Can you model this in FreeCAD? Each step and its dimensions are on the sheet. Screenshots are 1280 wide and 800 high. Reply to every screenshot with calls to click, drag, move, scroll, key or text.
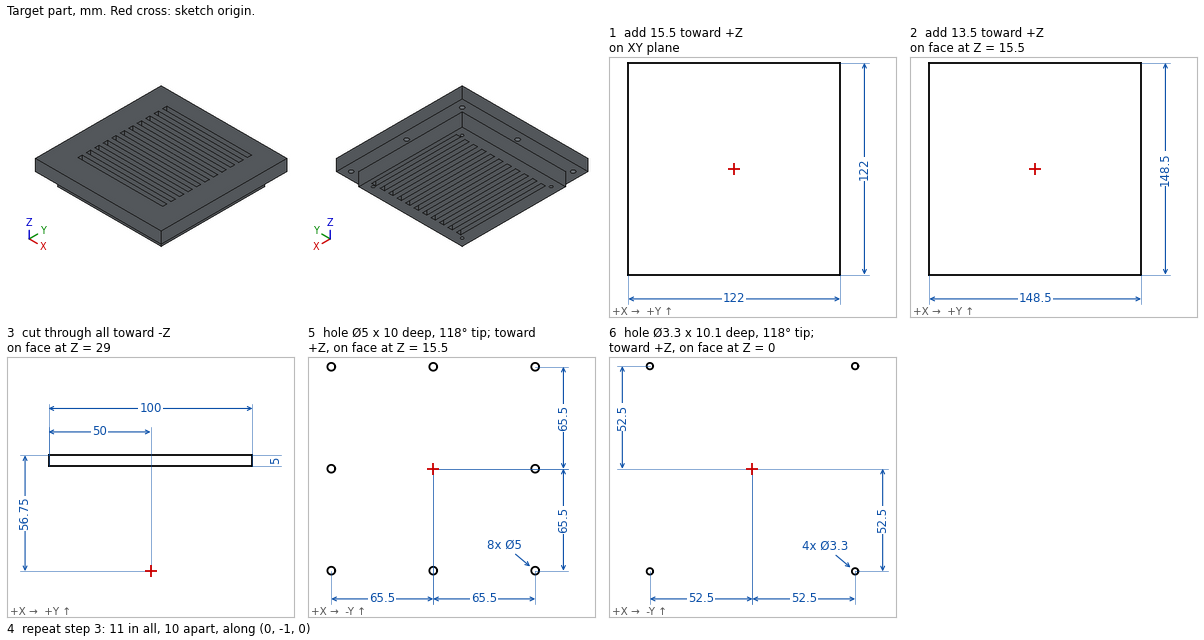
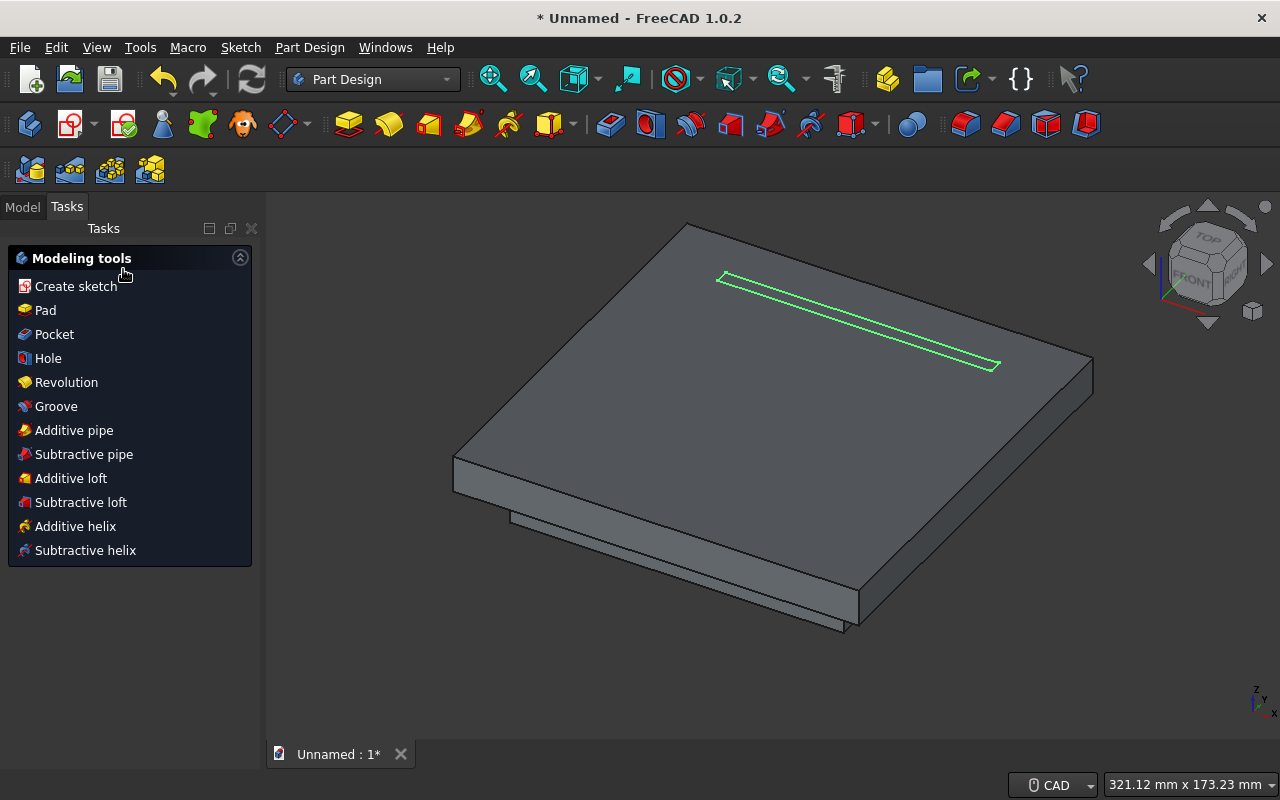
click(612, 124)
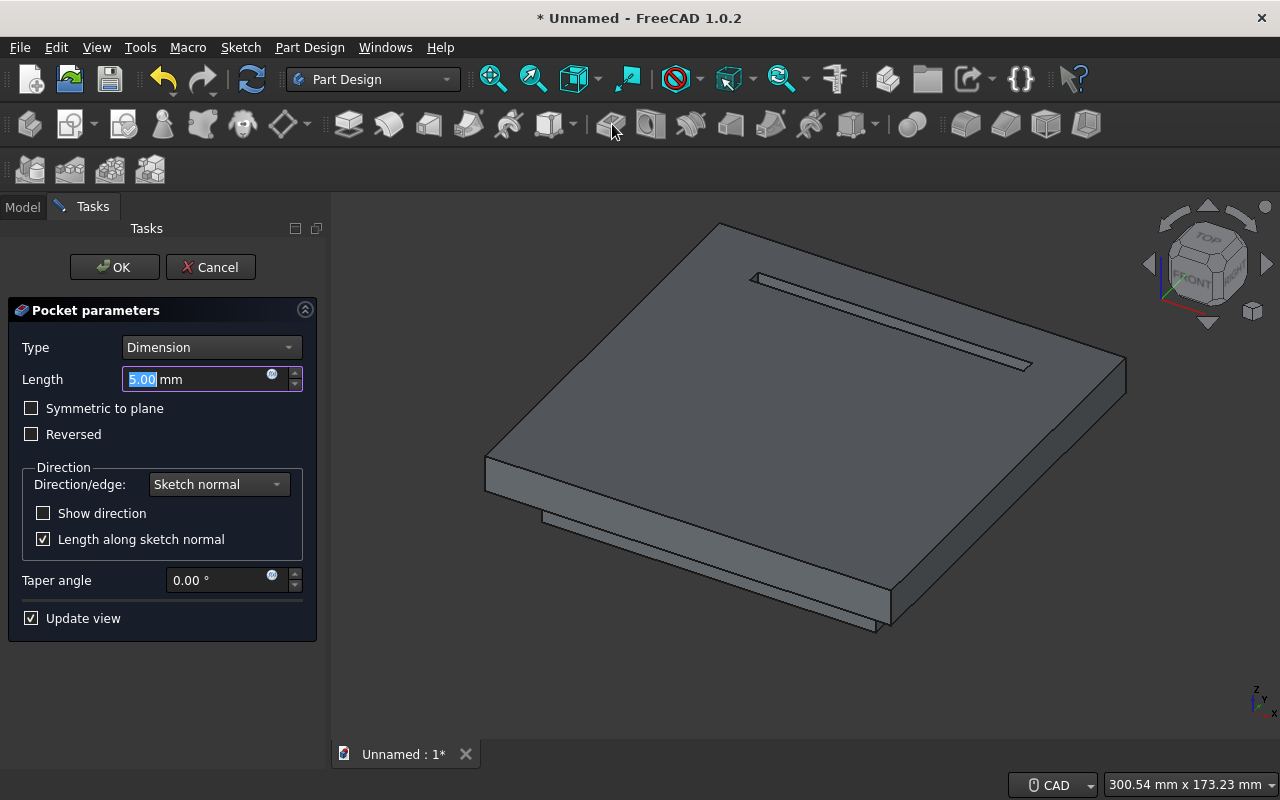
click(212, 348)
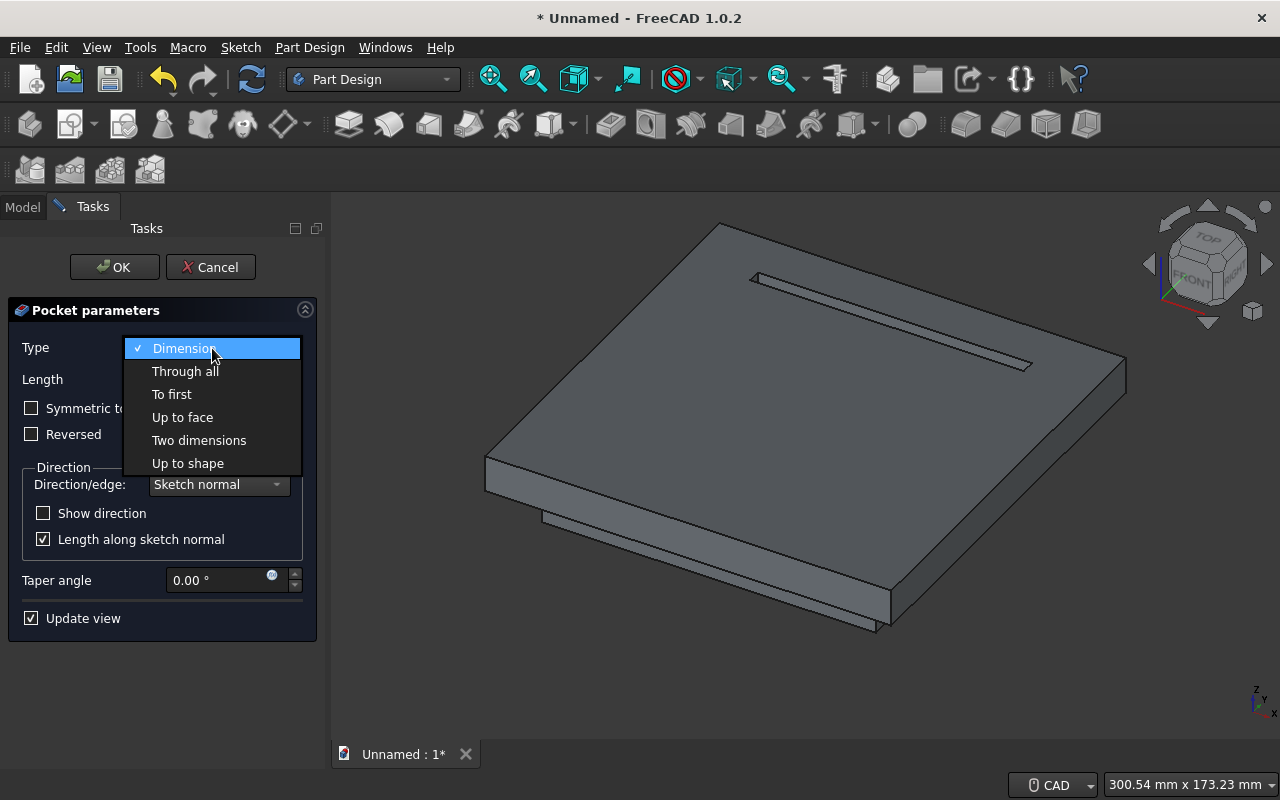
click(212, 372)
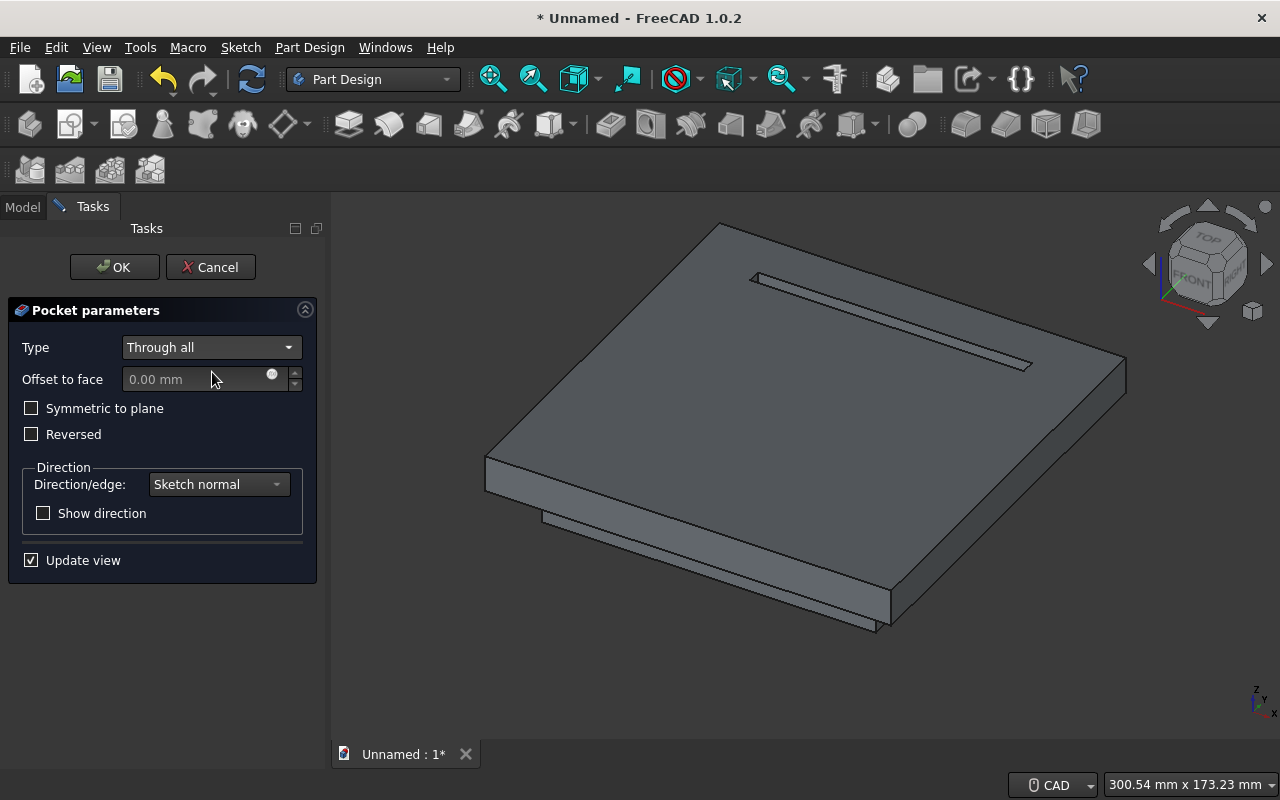
click(115, 267)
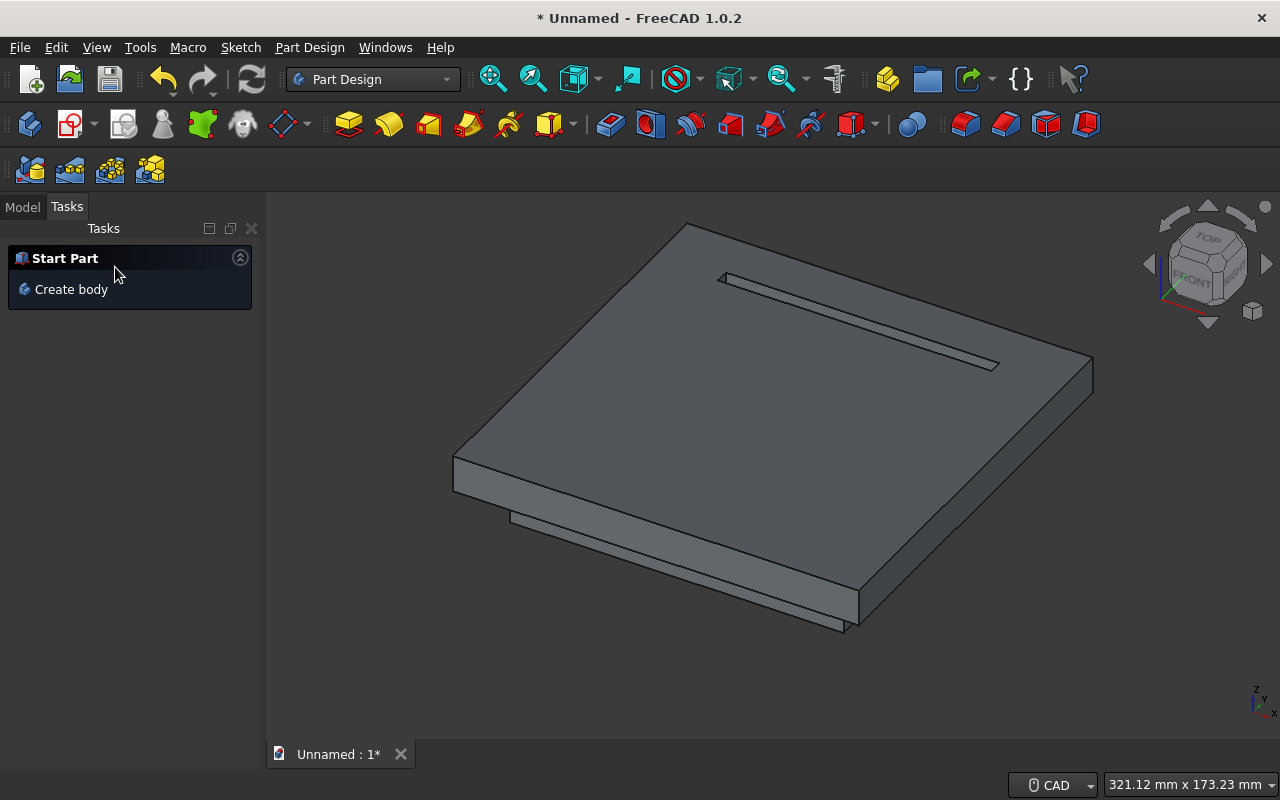
click(23, 206)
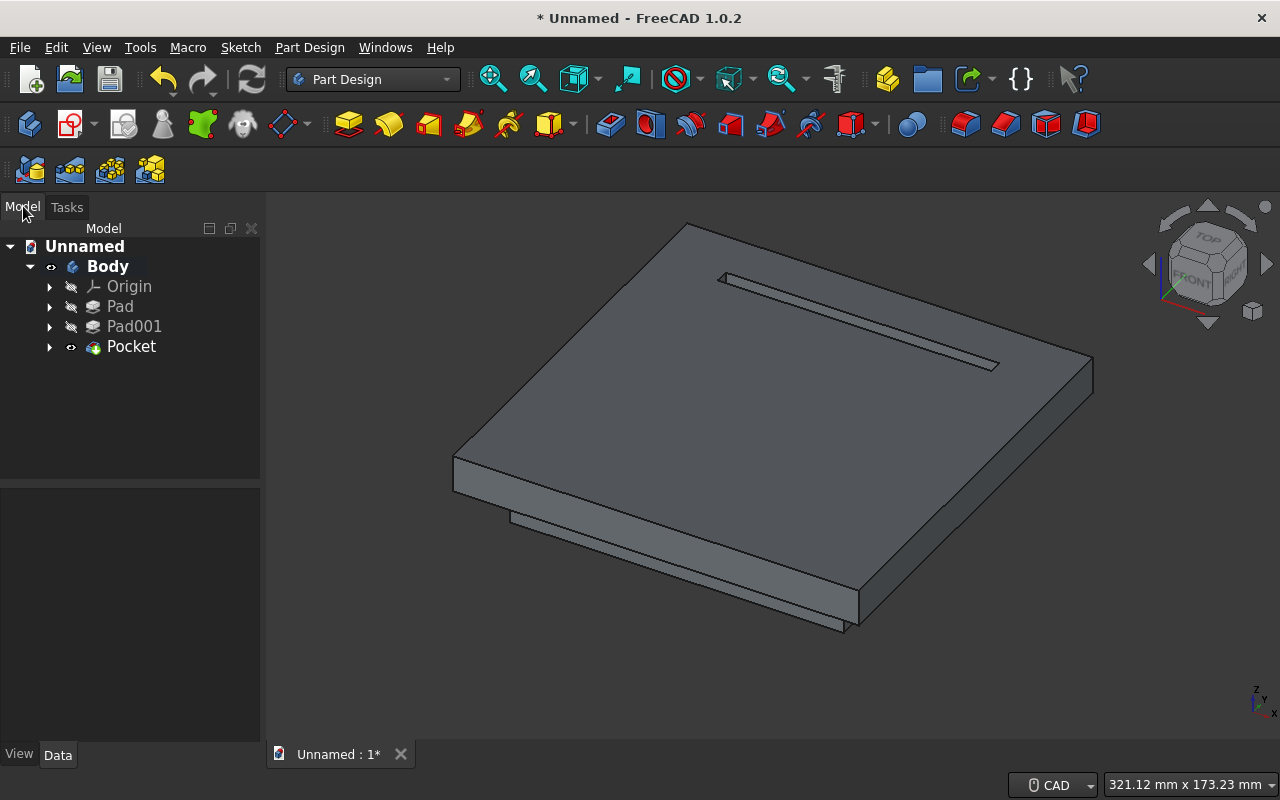
click(116, 347)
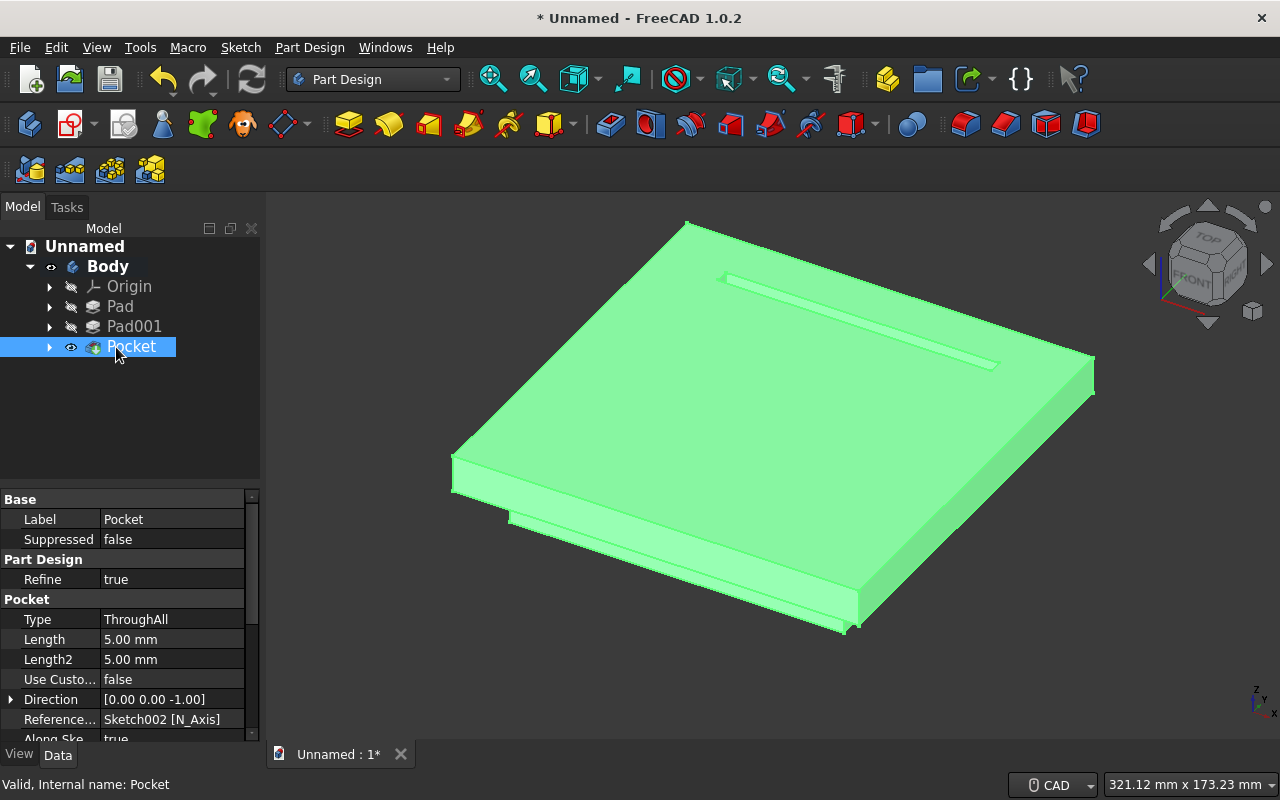
click(70, 170)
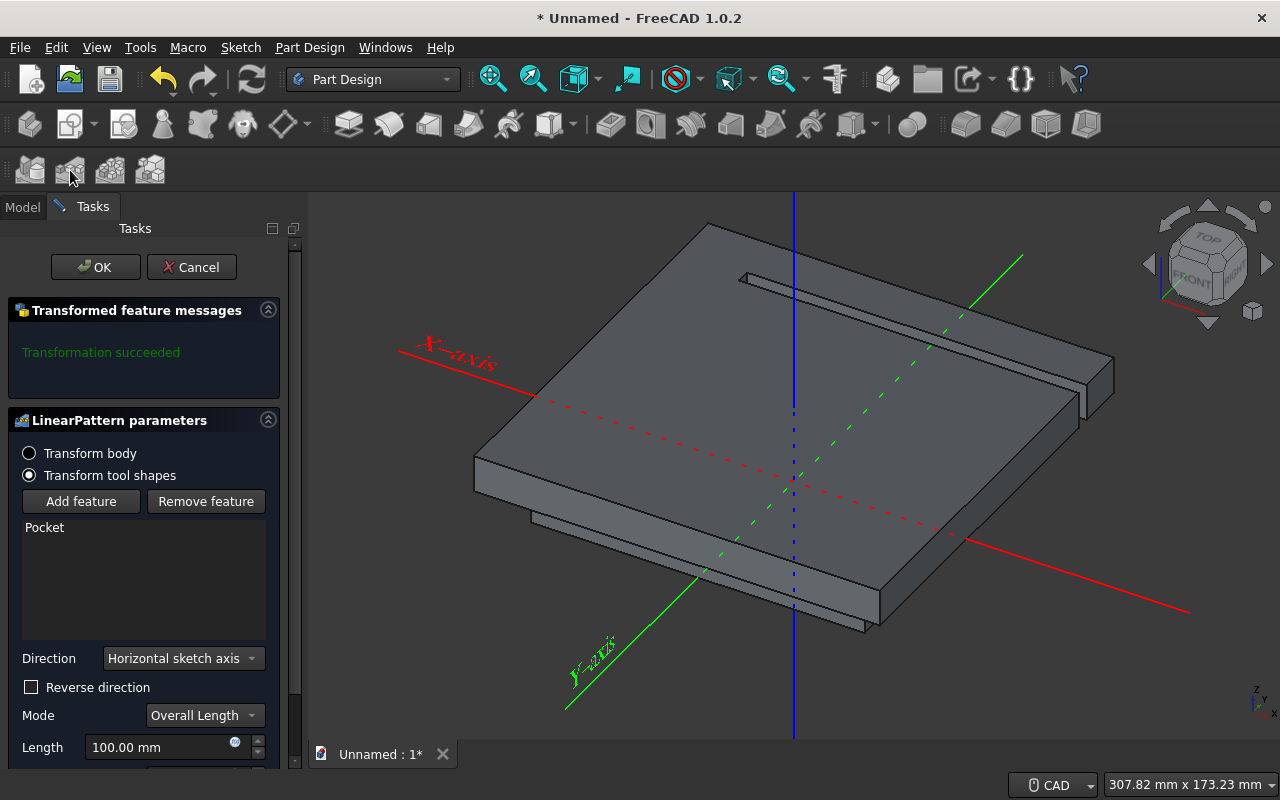
click(184, 658)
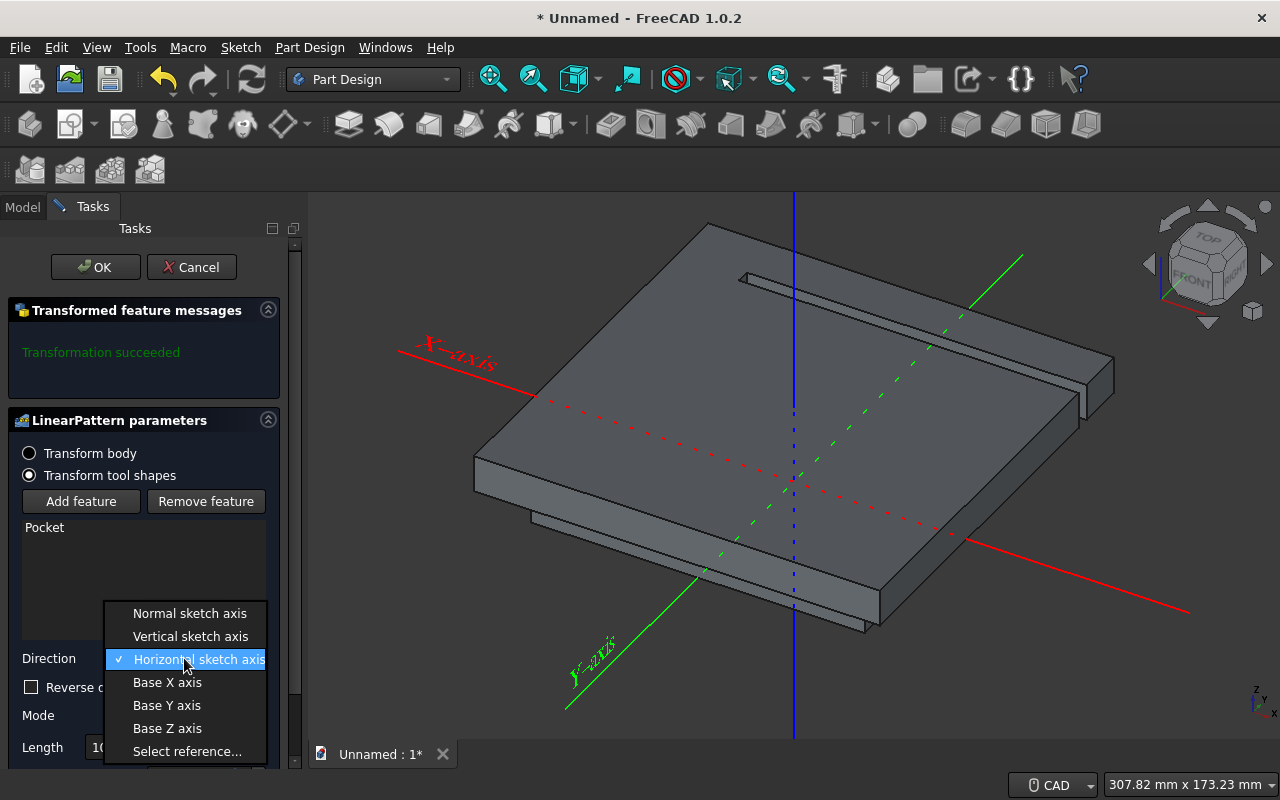
click(184, 706)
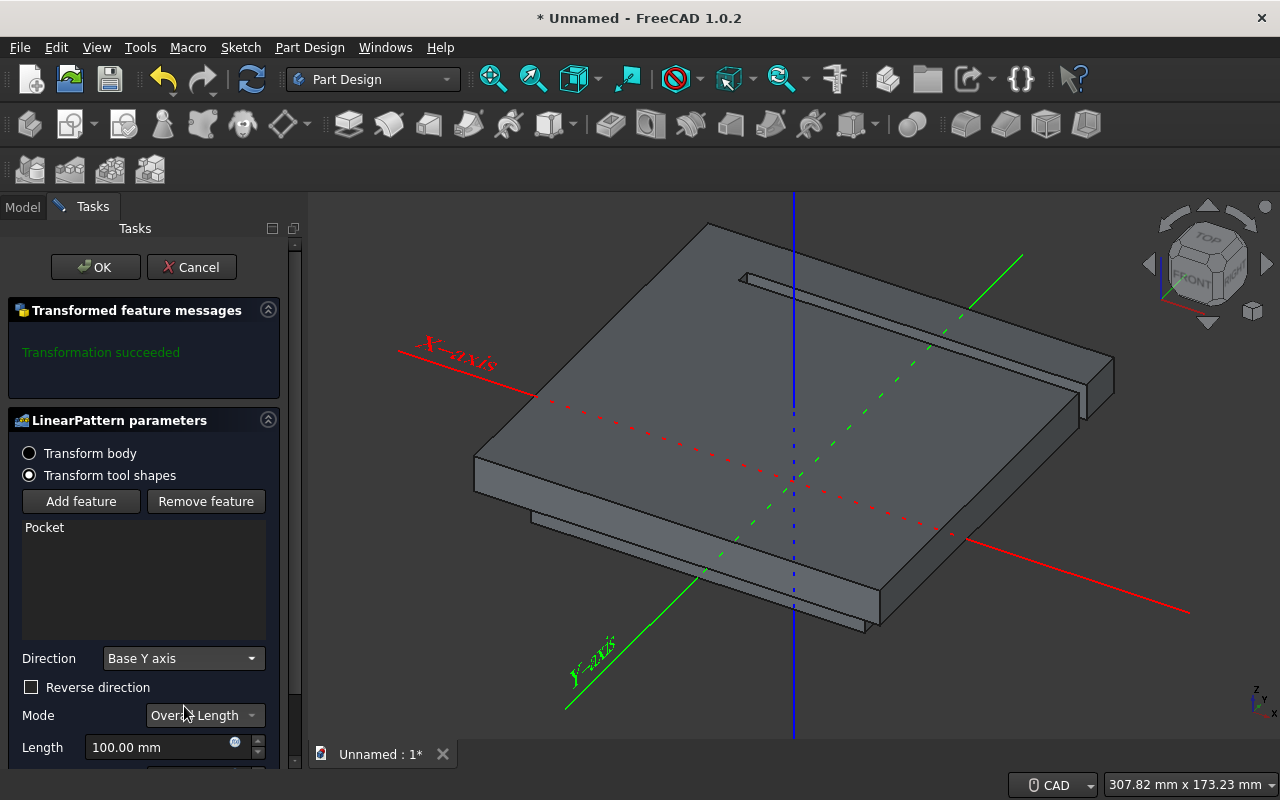
click(206, 716)